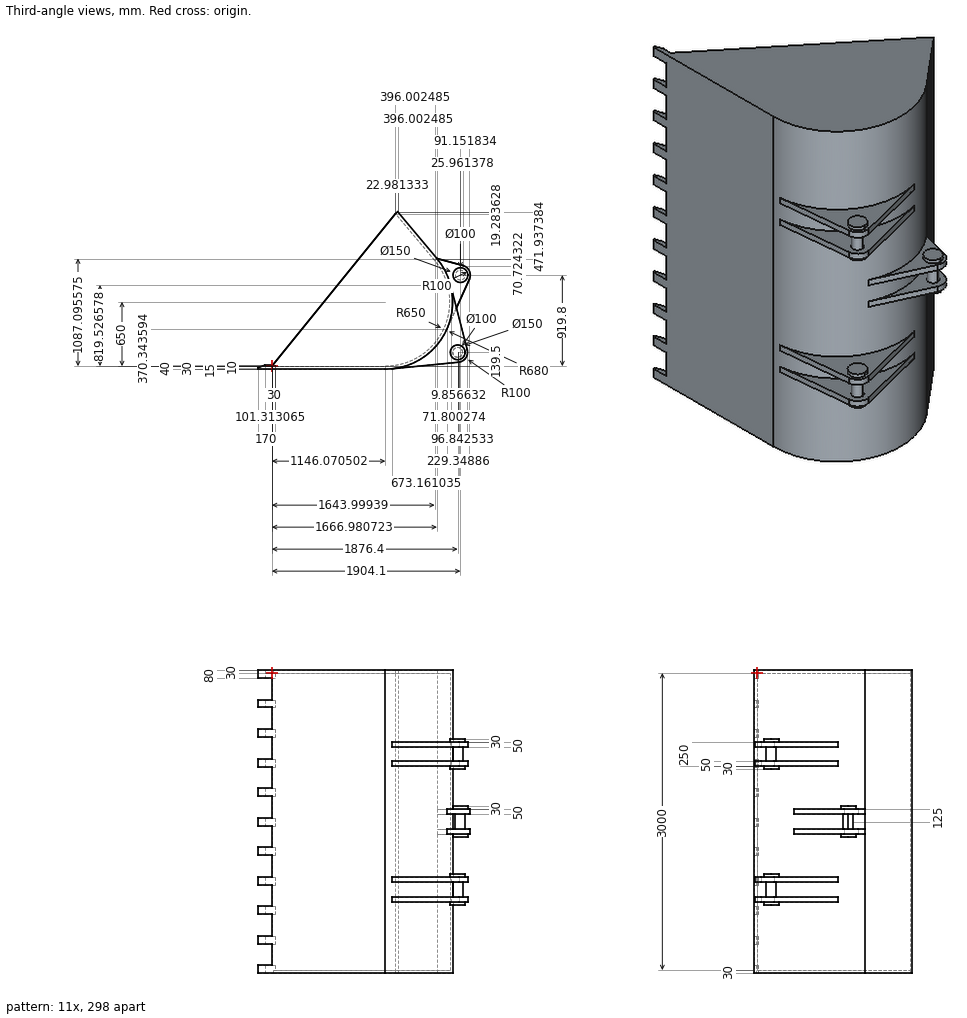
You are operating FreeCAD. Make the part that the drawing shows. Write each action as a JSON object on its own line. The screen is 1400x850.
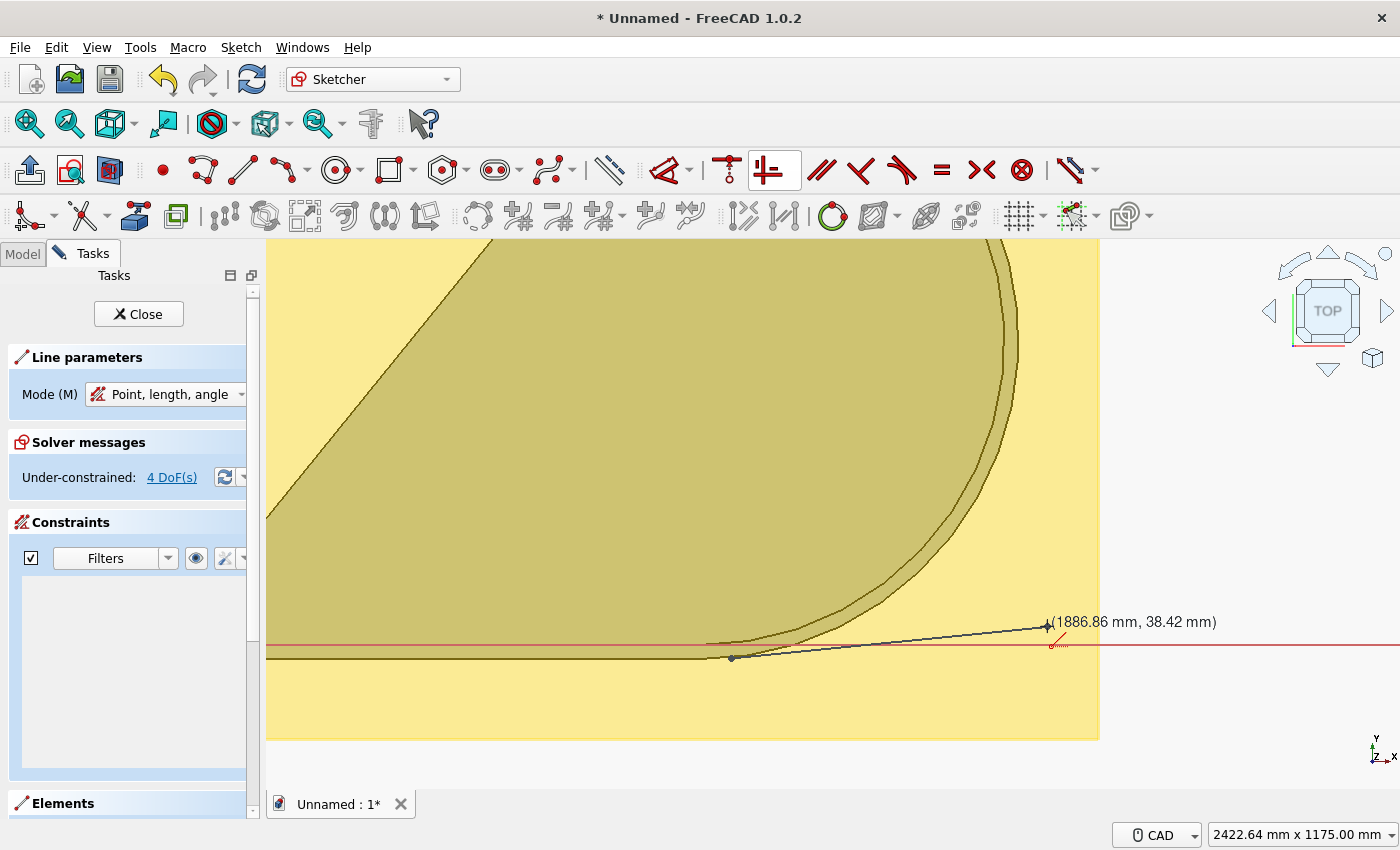
{"action": "left_click", "coordinate": [1087, 568]}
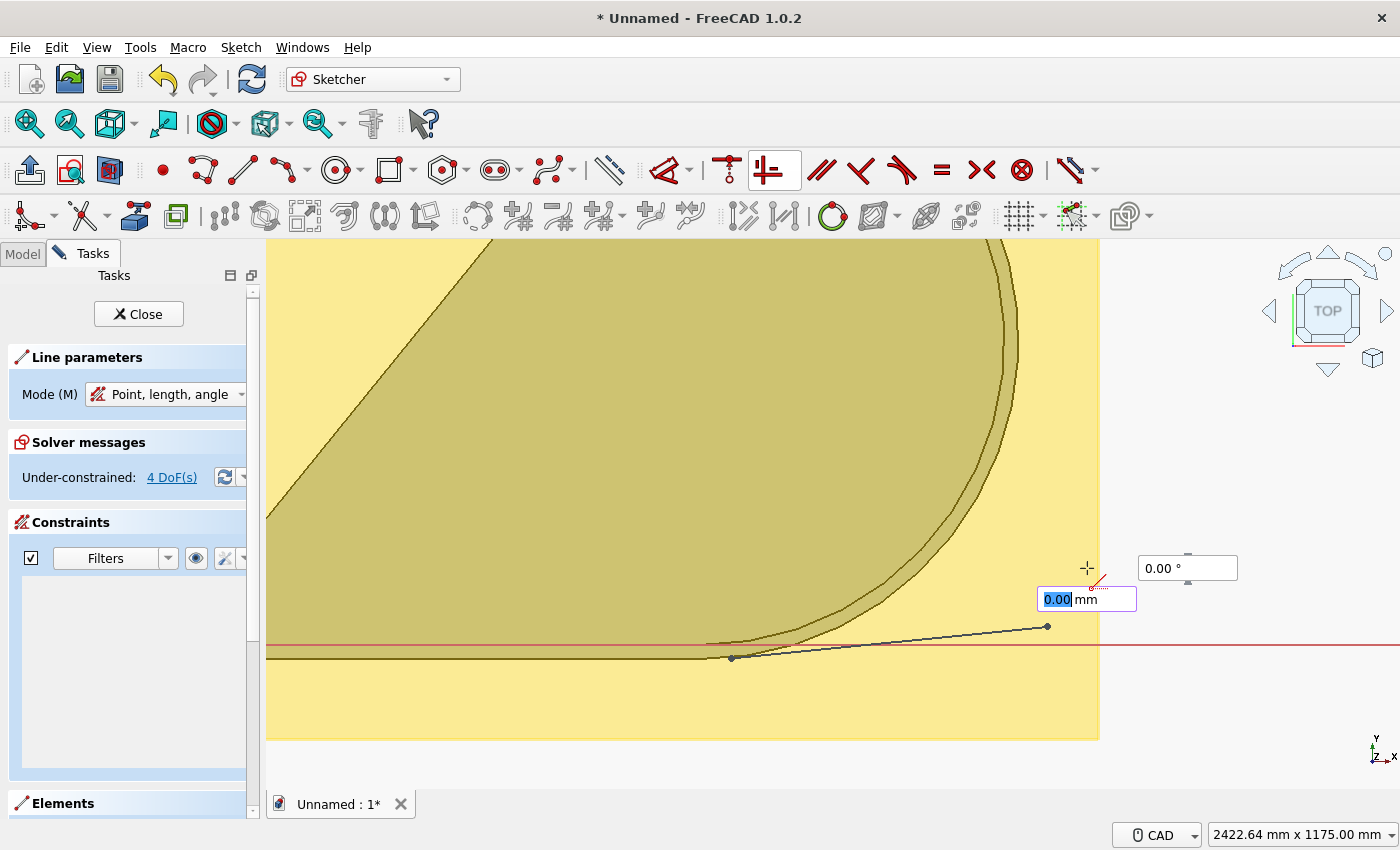
{"action": "scroll", "coordinate": [1047, 625], "scroll_direction": "down", "scroll_amount": 2}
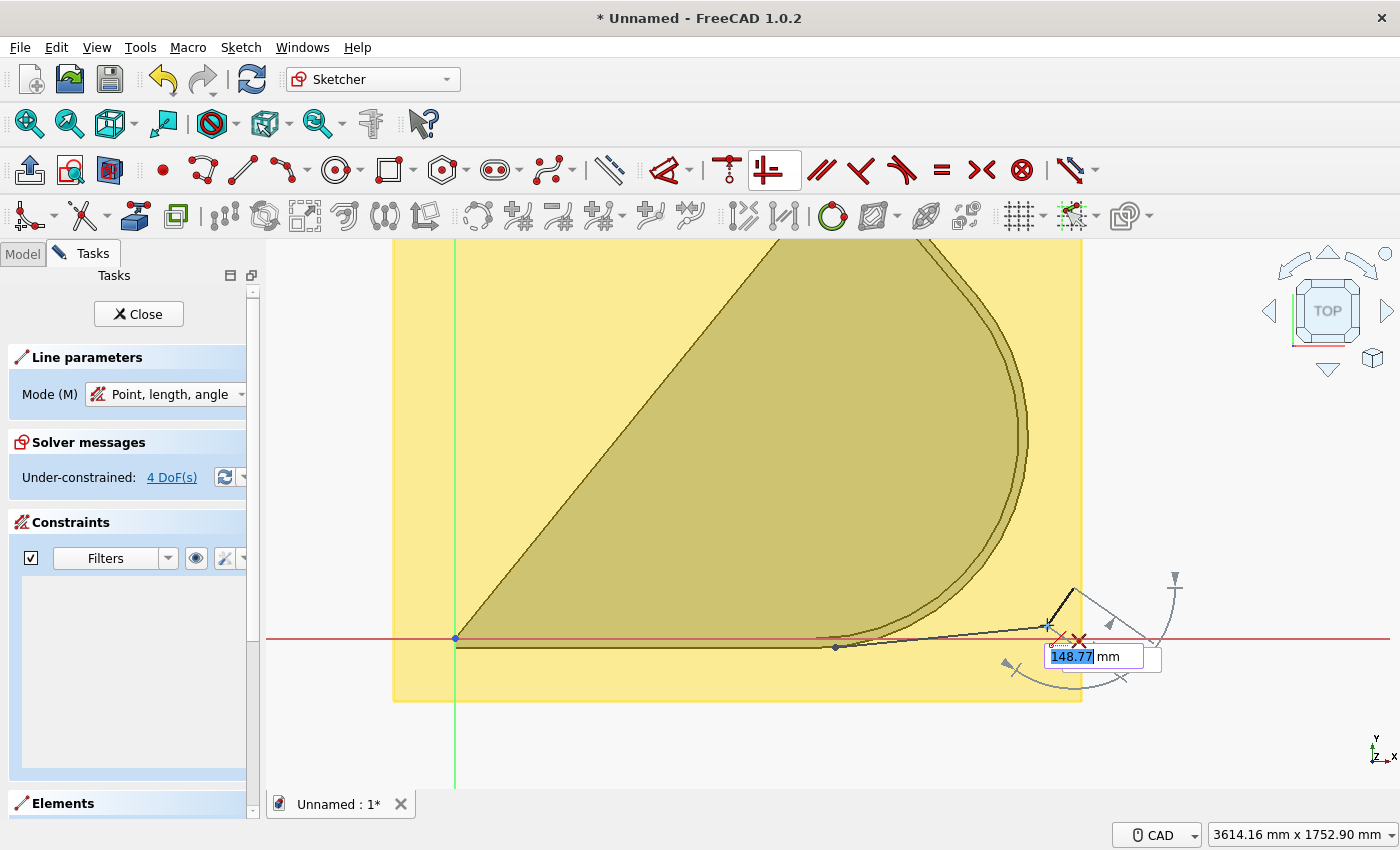
{"action": "left_click", "coordinate": [1021, 381]}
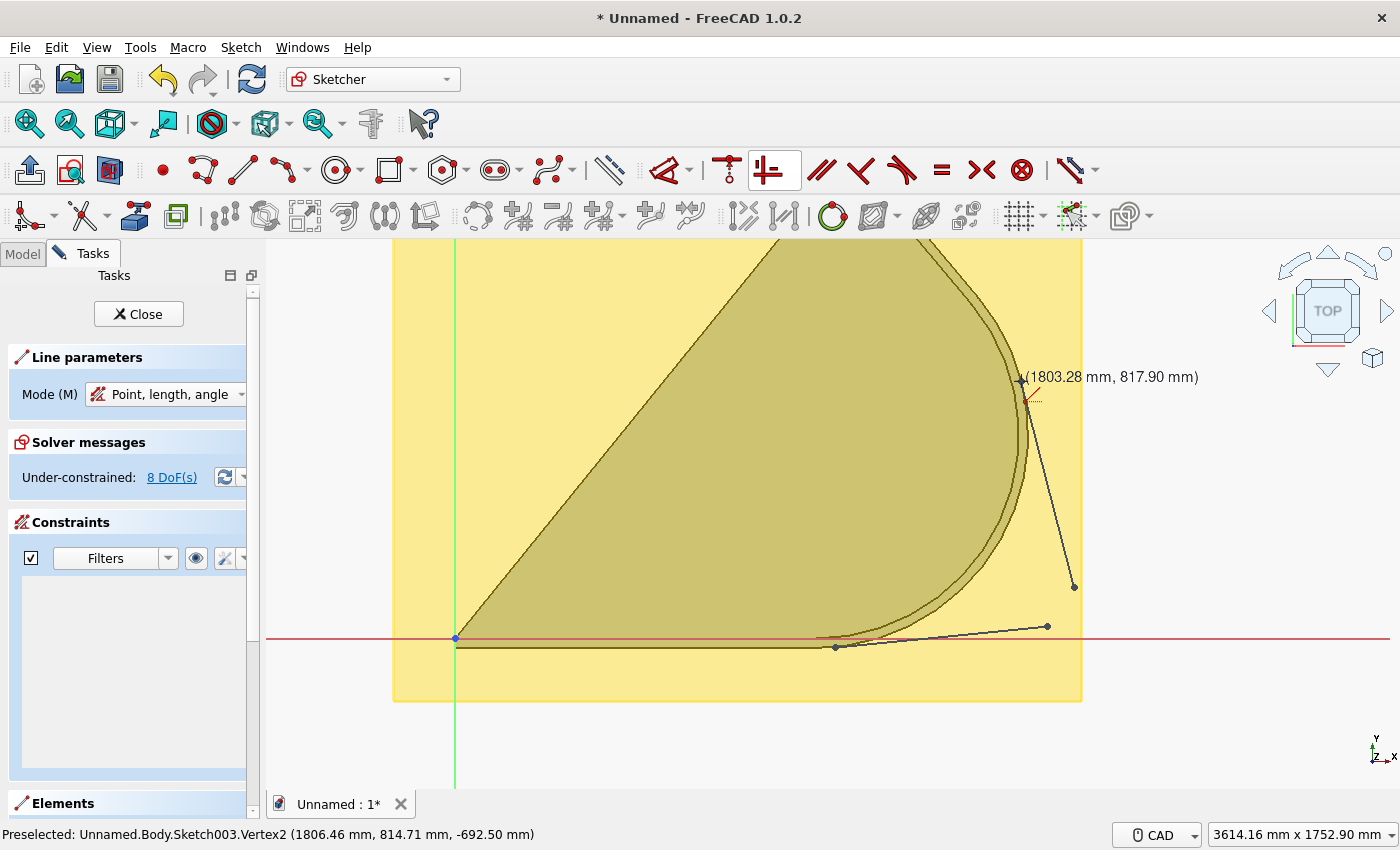
{"action": "left_click", "coordinate": [284, 170]}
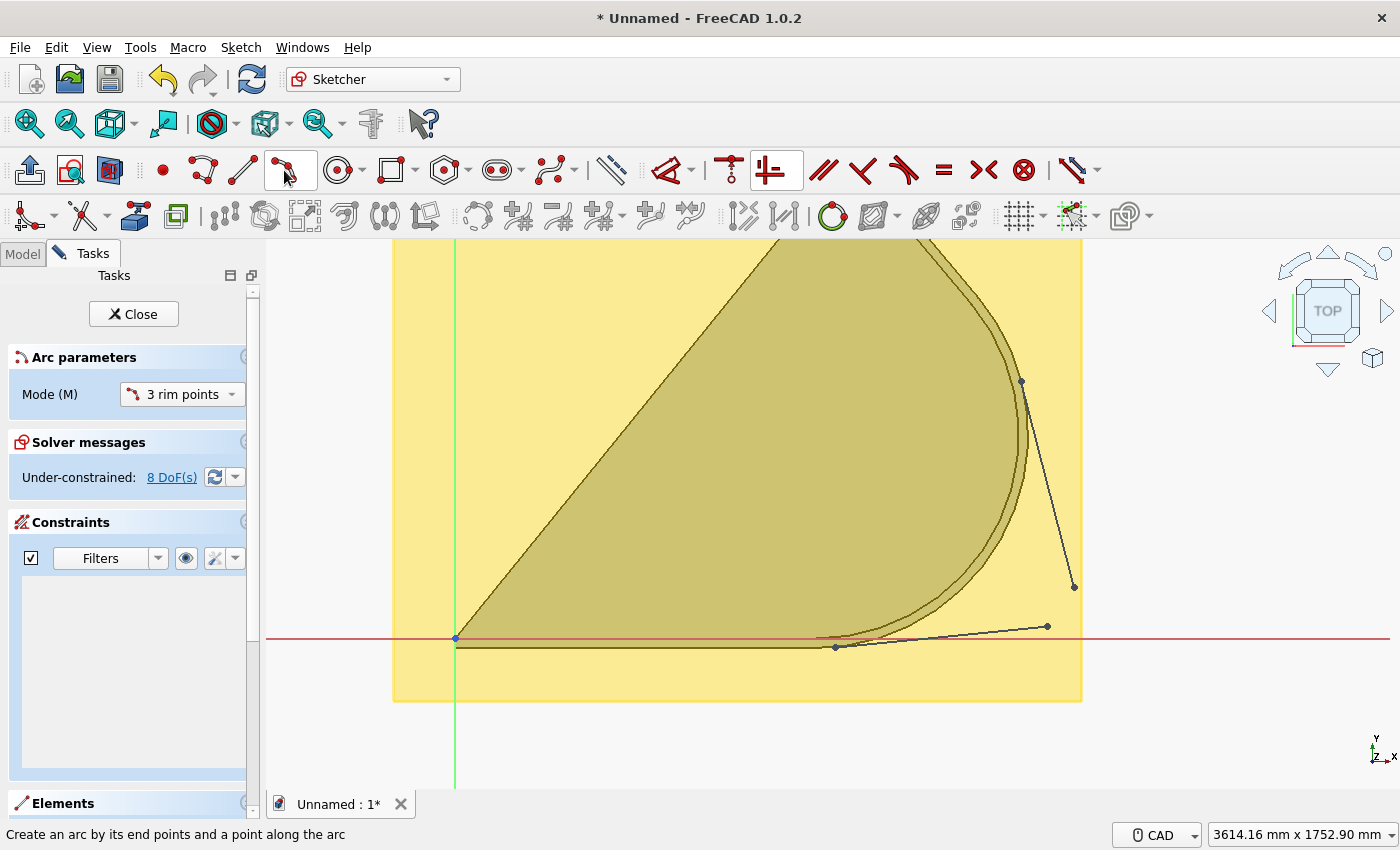
{"action": "scroll", "coordinate": [1047, 626], "scroll_direction": "up", "scroll_amount": 2}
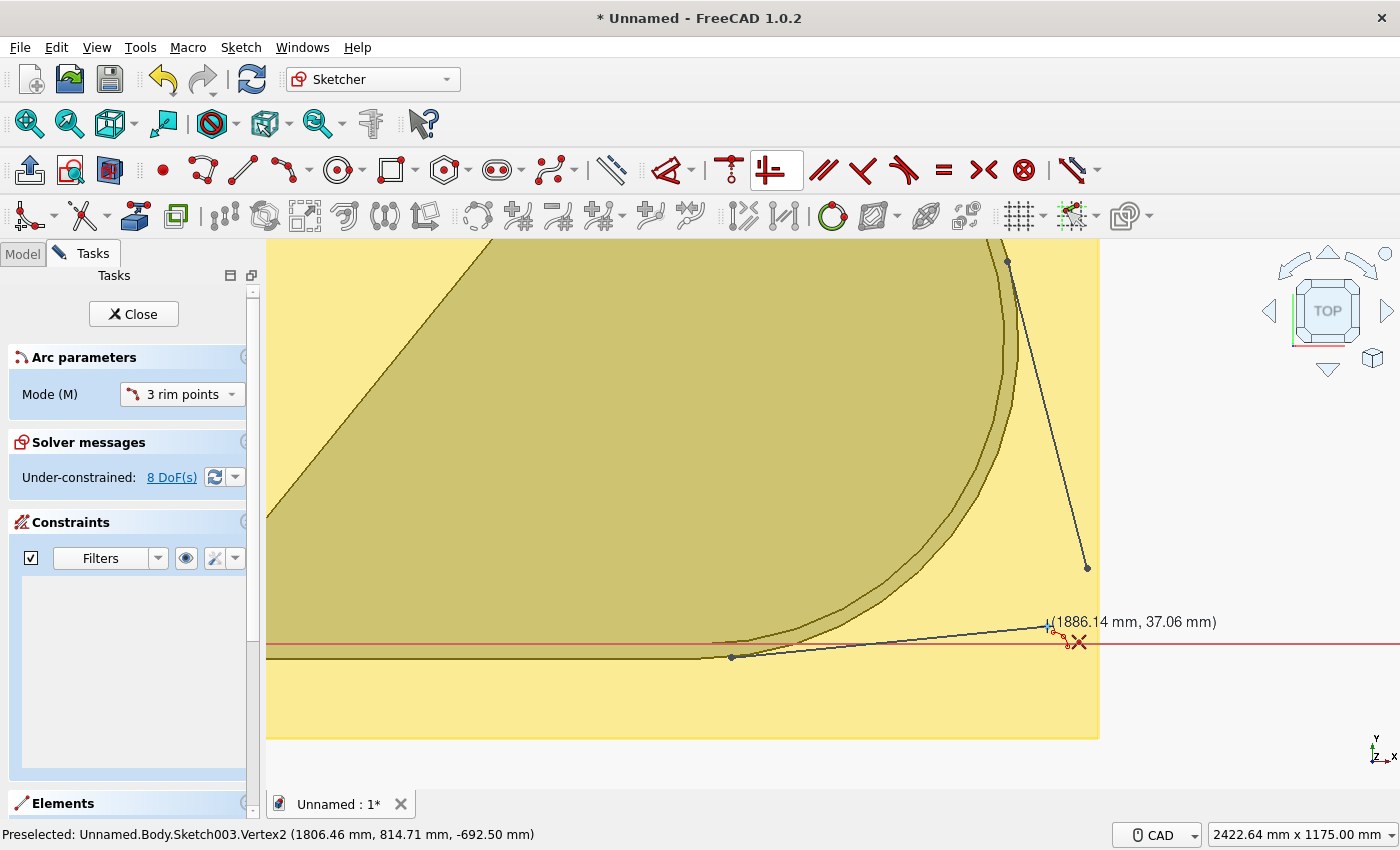
{"action": "left_click", "coordinate": [1047, 627]}
{"action": "left_click", "coordinate": [1087, 569]}
{"action": "left_click", "coordinate": [1080, 606]}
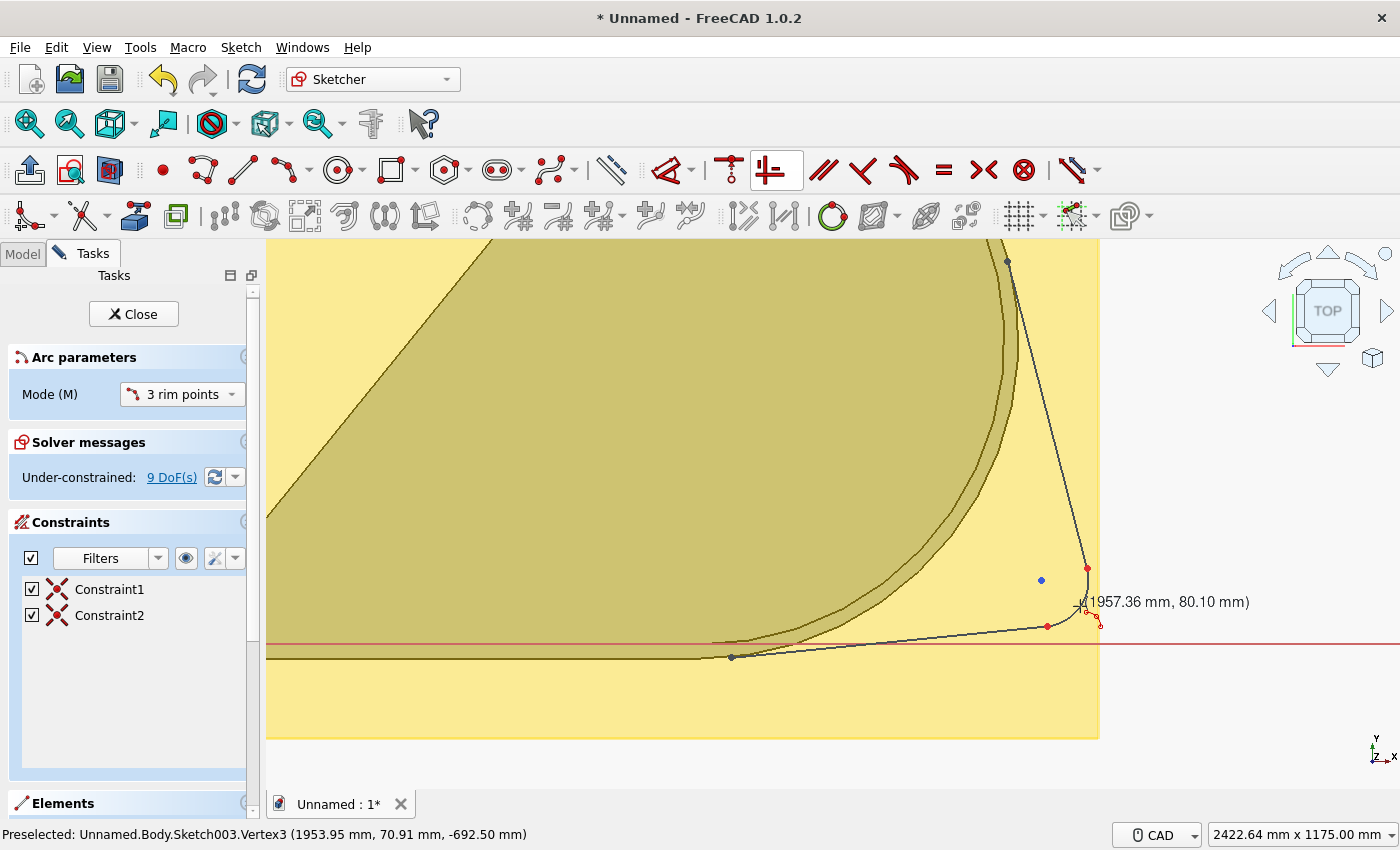
{"action": "scroll", "coordinate": [1047, 626], "scroll_direction": "down", "scroll_amount": 2}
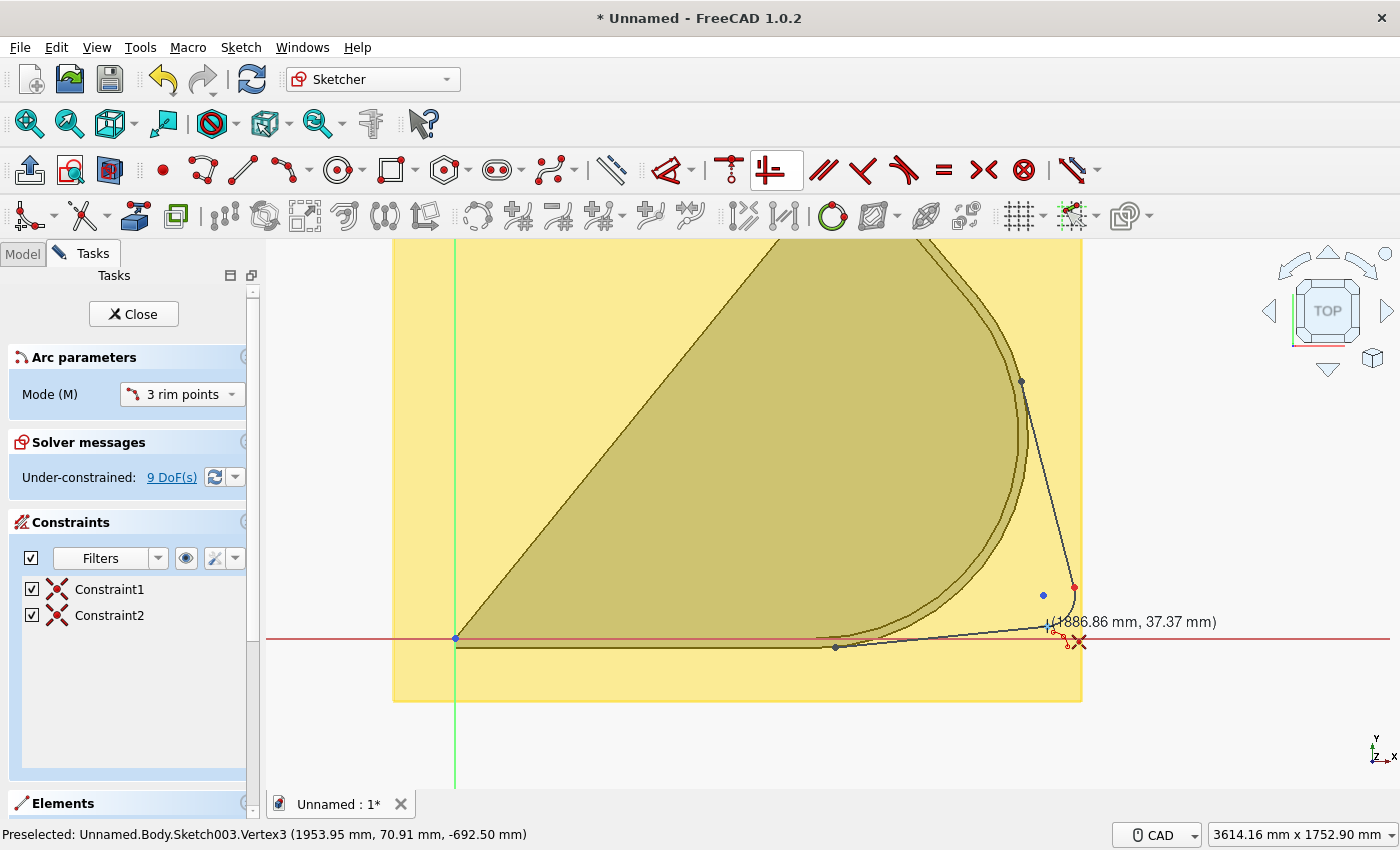
{"action": "left_click", "coordinate": [1021, 382]}